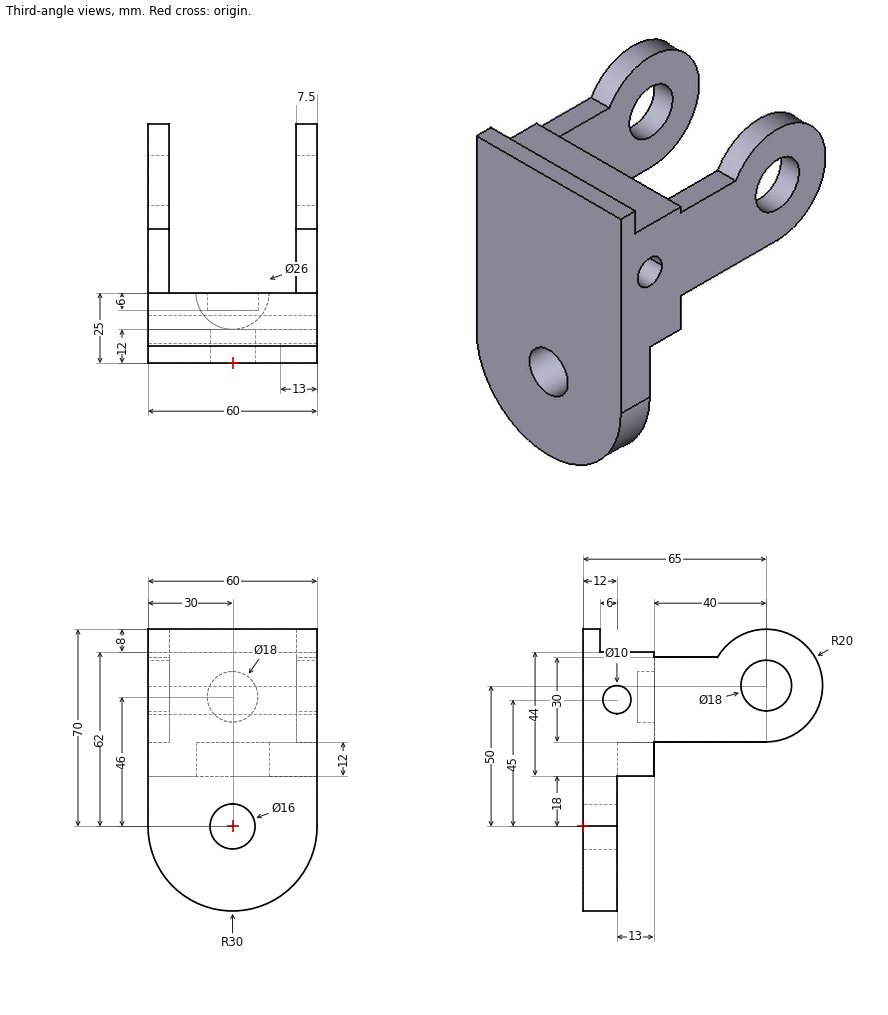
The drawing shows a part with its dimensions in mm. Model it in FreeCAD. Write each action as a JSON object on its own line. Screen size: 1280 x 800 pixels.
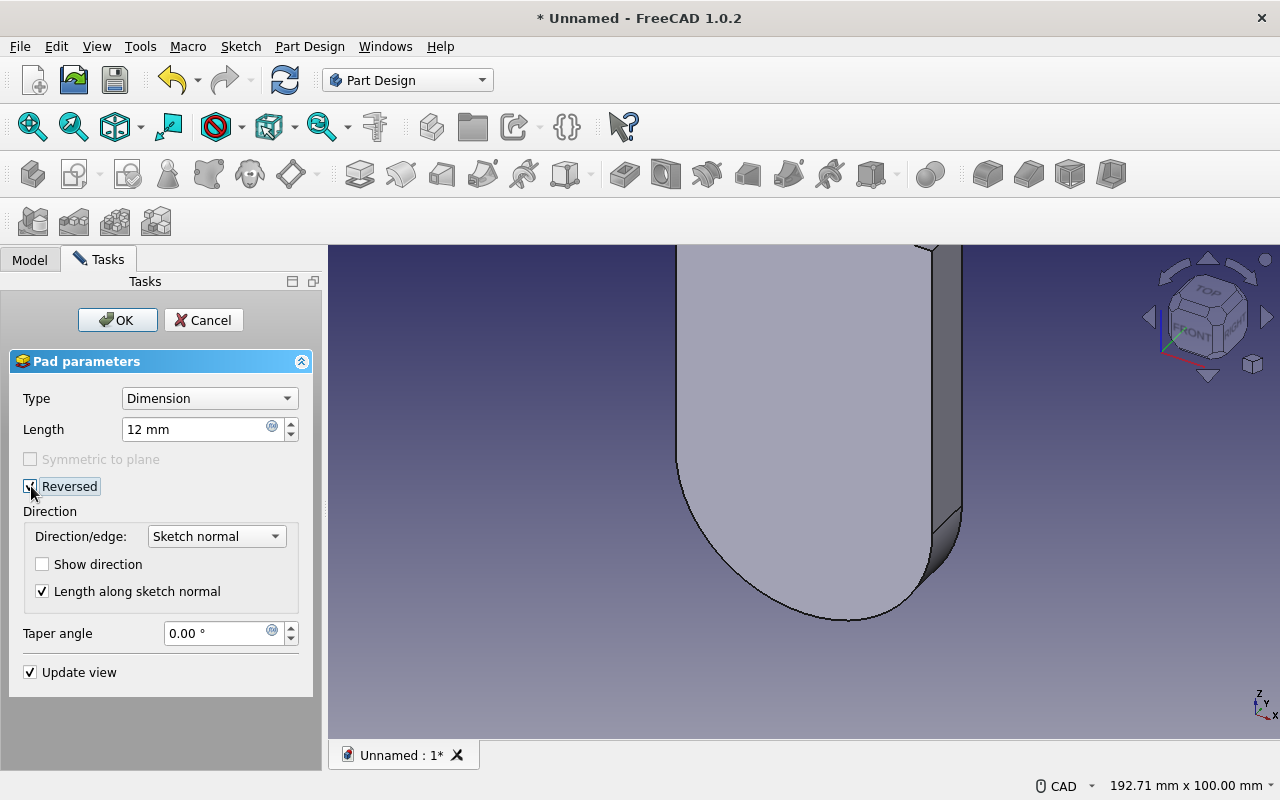
{"action": "left_click", "coordinate": [118, 320]}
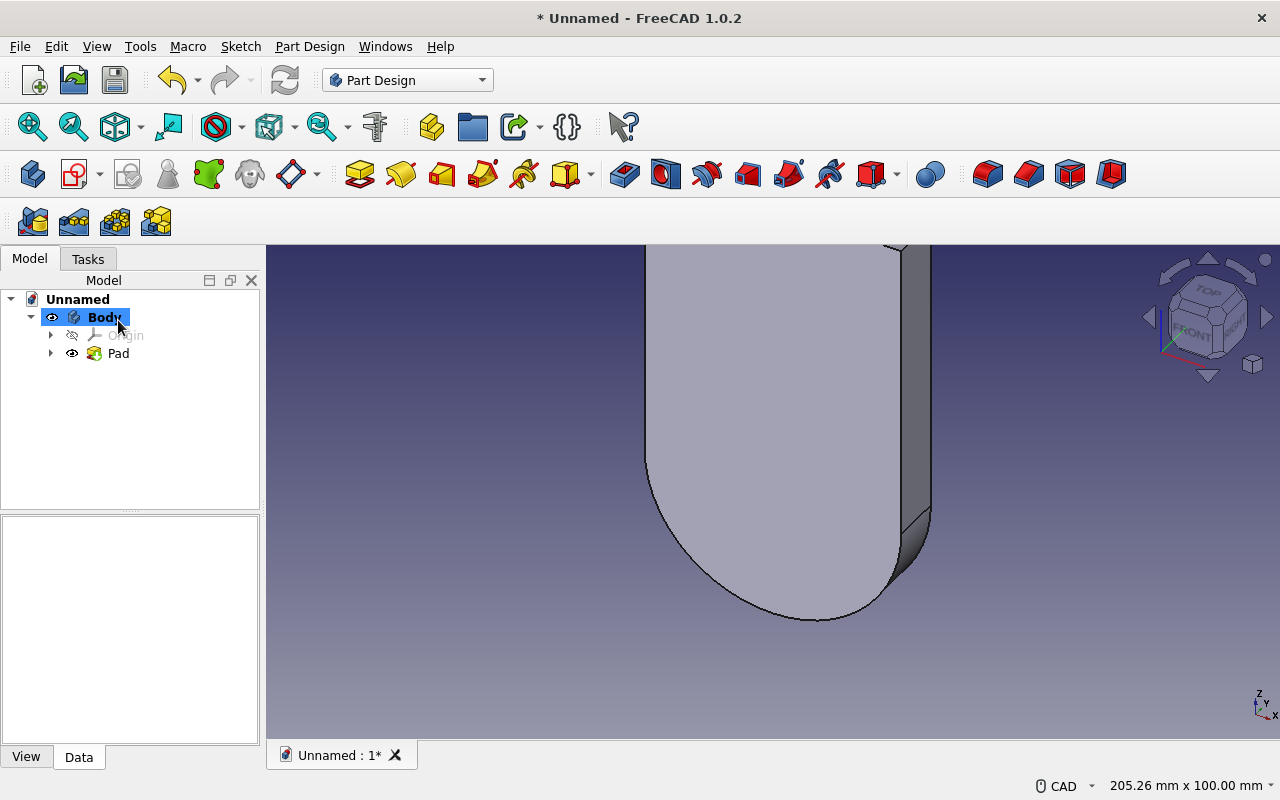
{"action": "key", "text": "v f"}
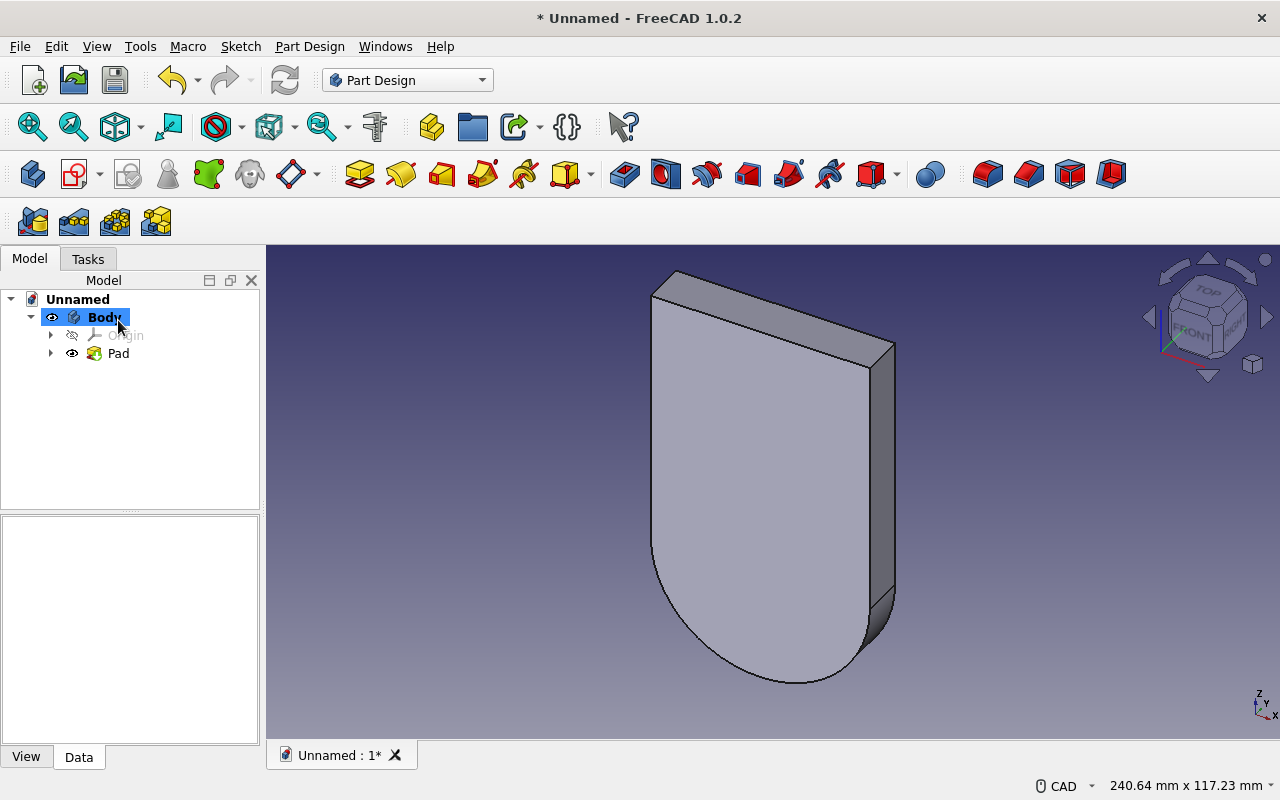
{"action": "key", "text": "4"}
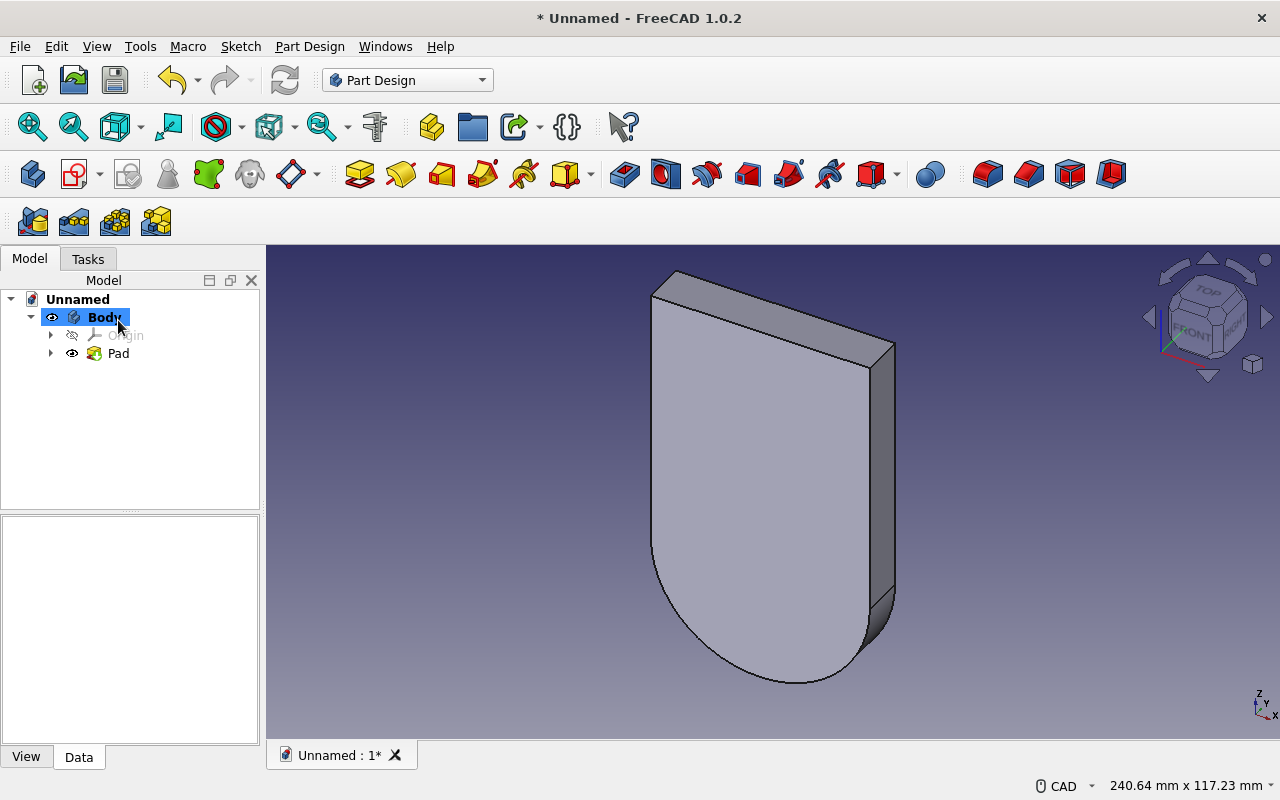
{"action": "left_click", "coordinate": [773, 431]}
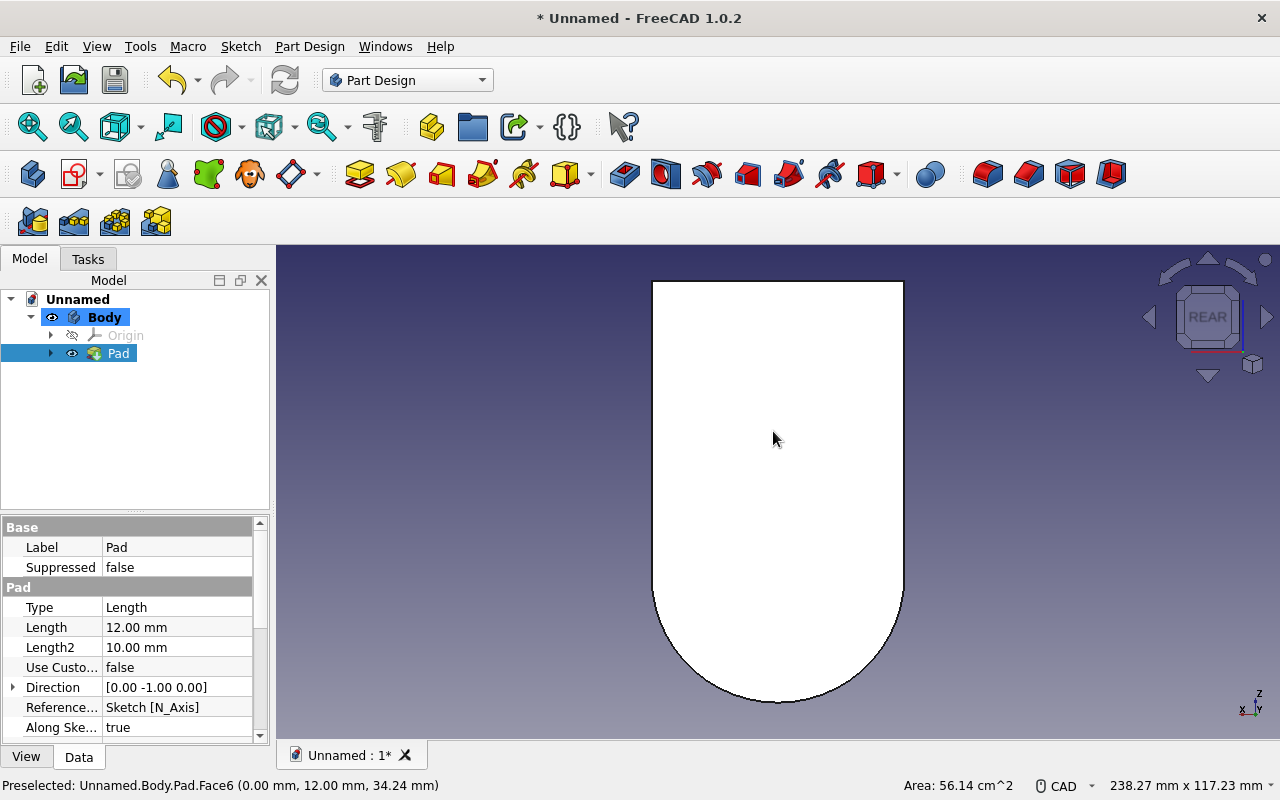
{"action": "left_click", "coordinate": [74, 174]}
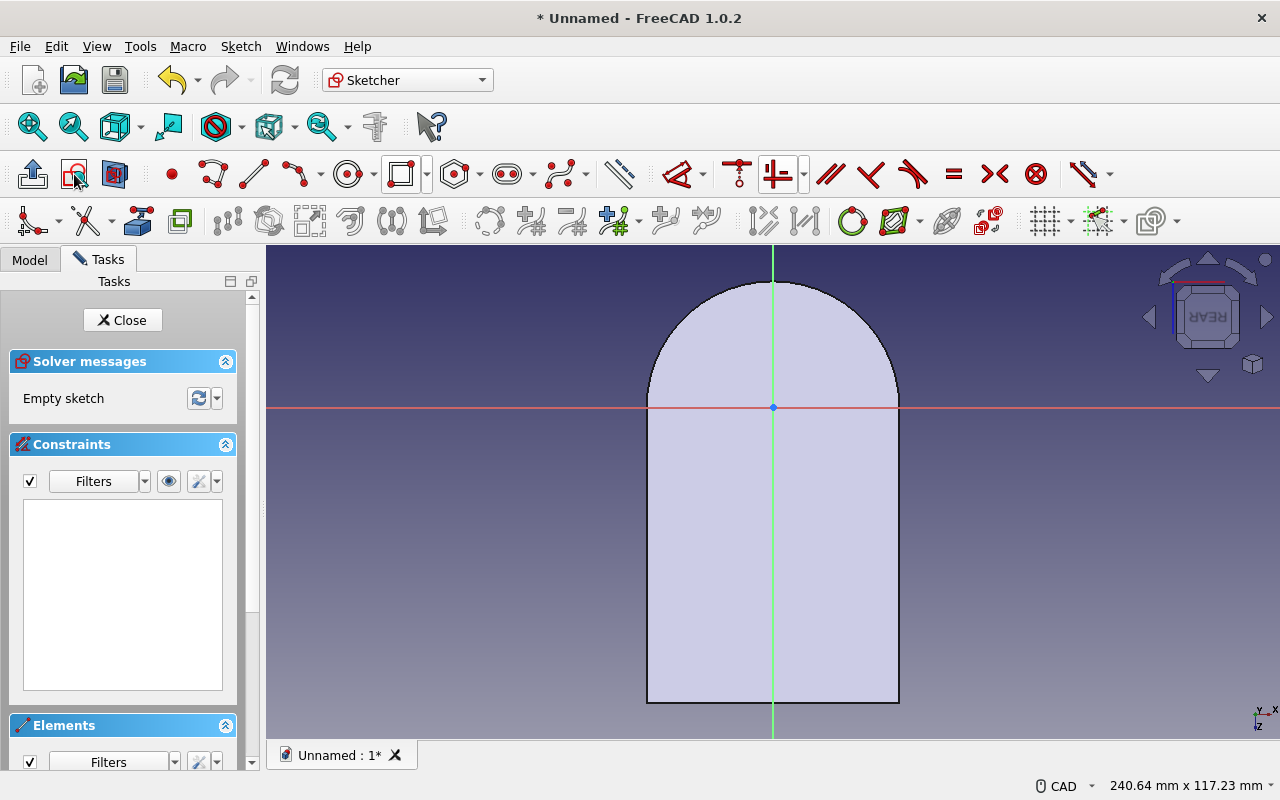
{"action": "scroll", "coordinate": [790, 386], "scroll_direction": "up", "scroll_amount": 8}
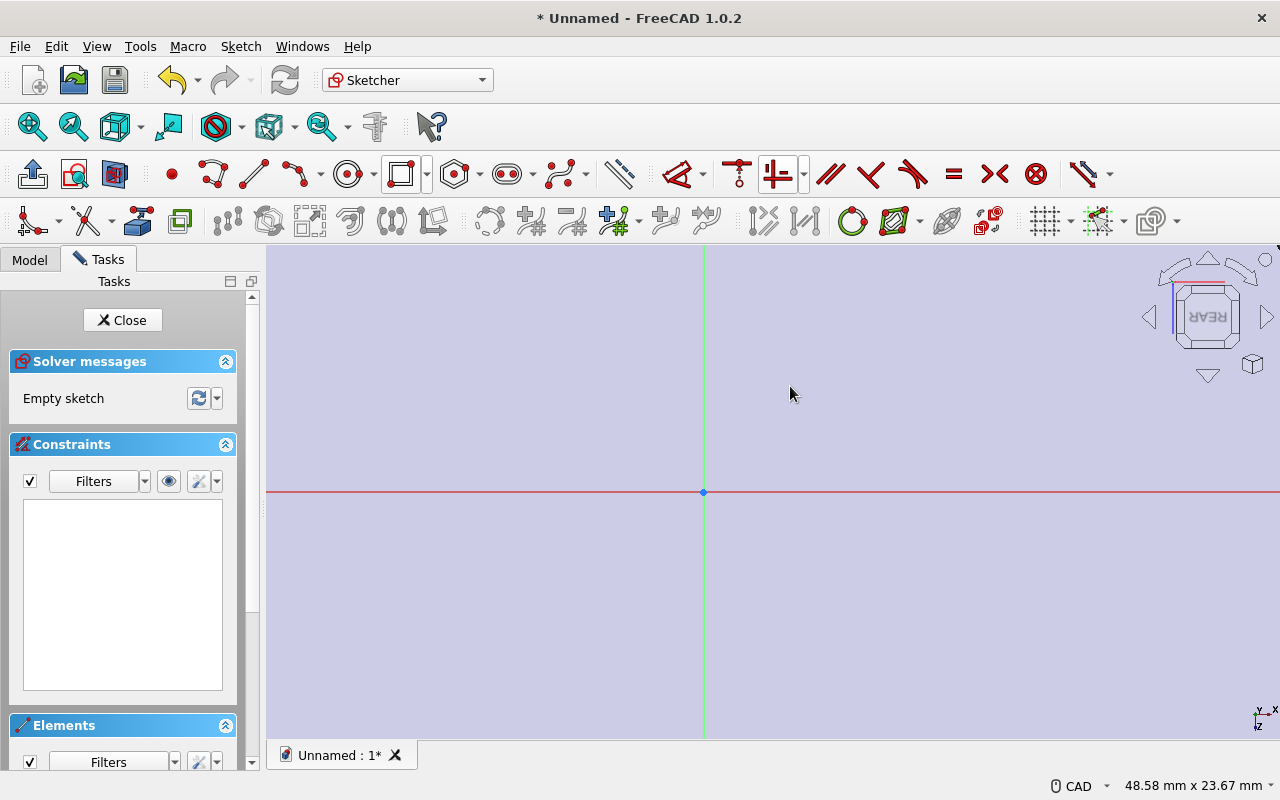
{"action": "key", "text": "g c"}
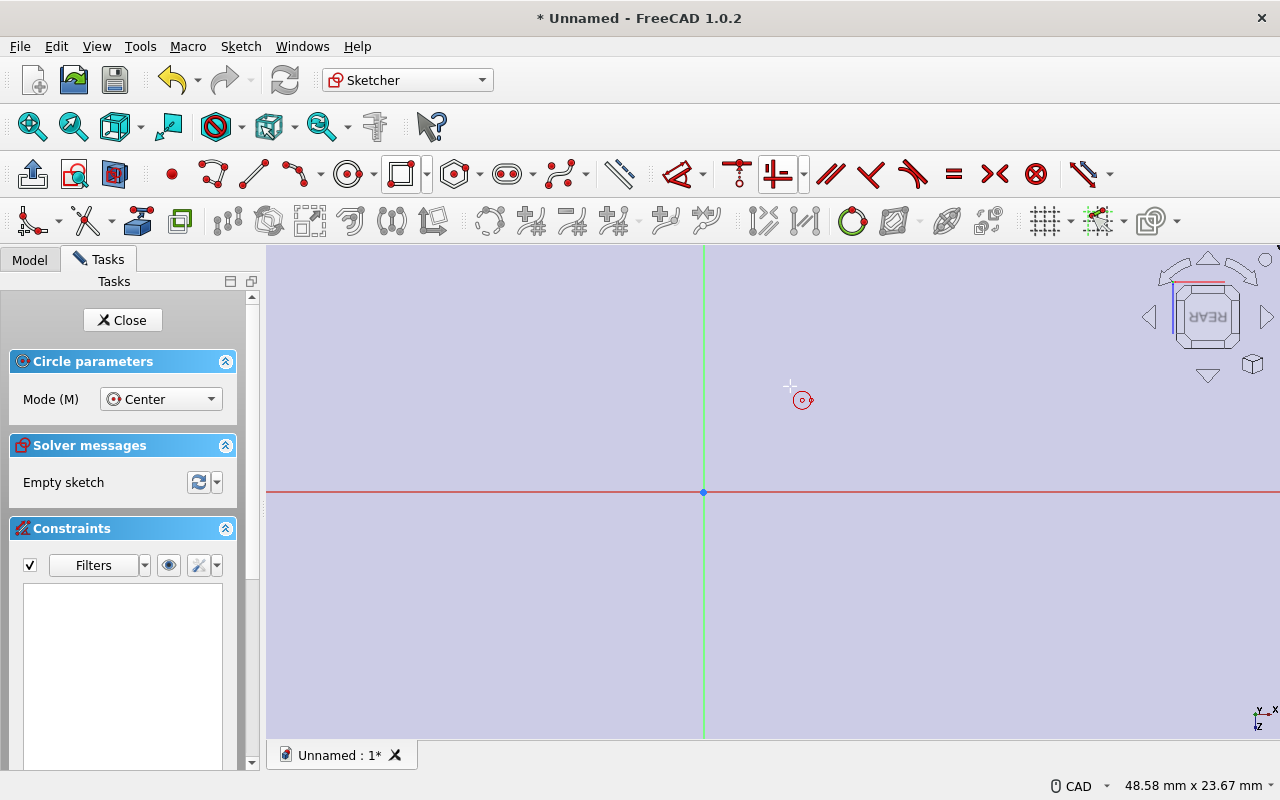
{"action": "left_click", "coordinate": [704, 492]}
{"action": "left_click", "coordinate": [822, 374]}
{"action": "key", "text": "Escape"}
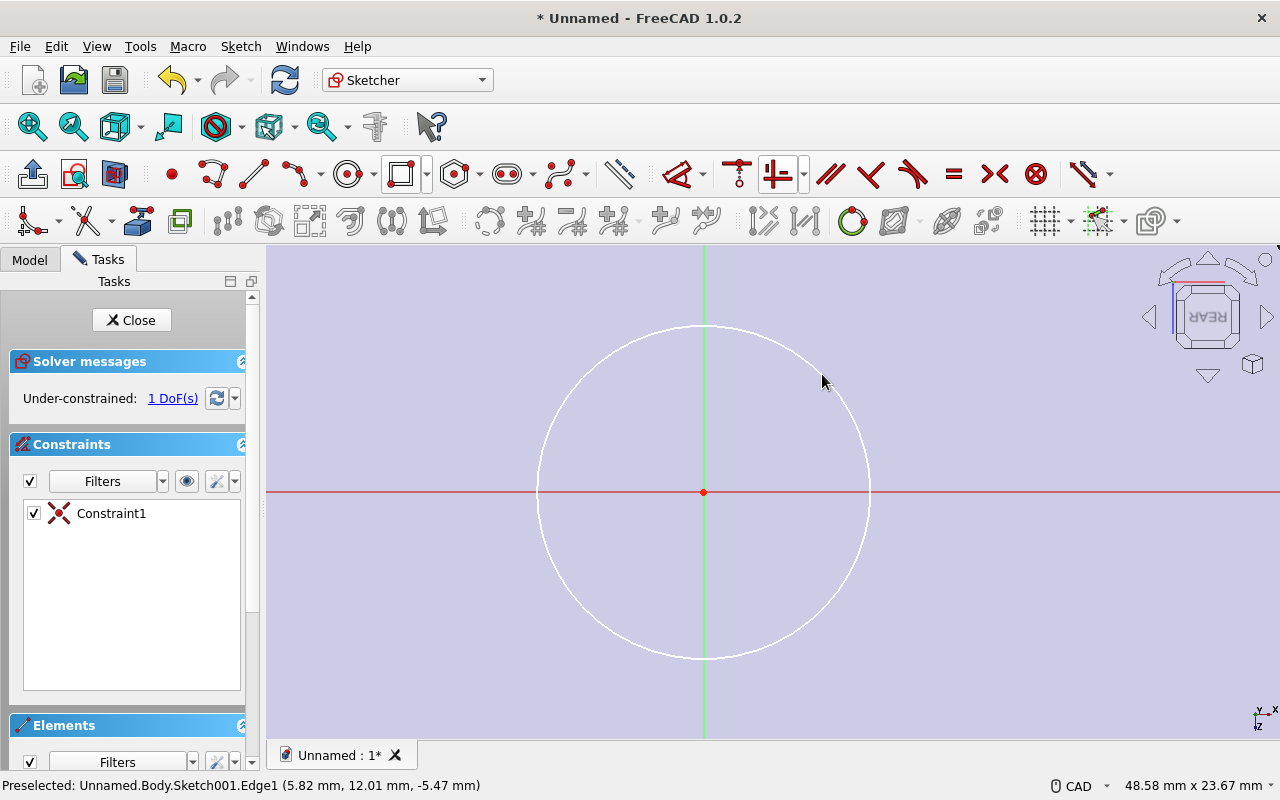
{"action": "left_click", "coordinate": [676, 174]}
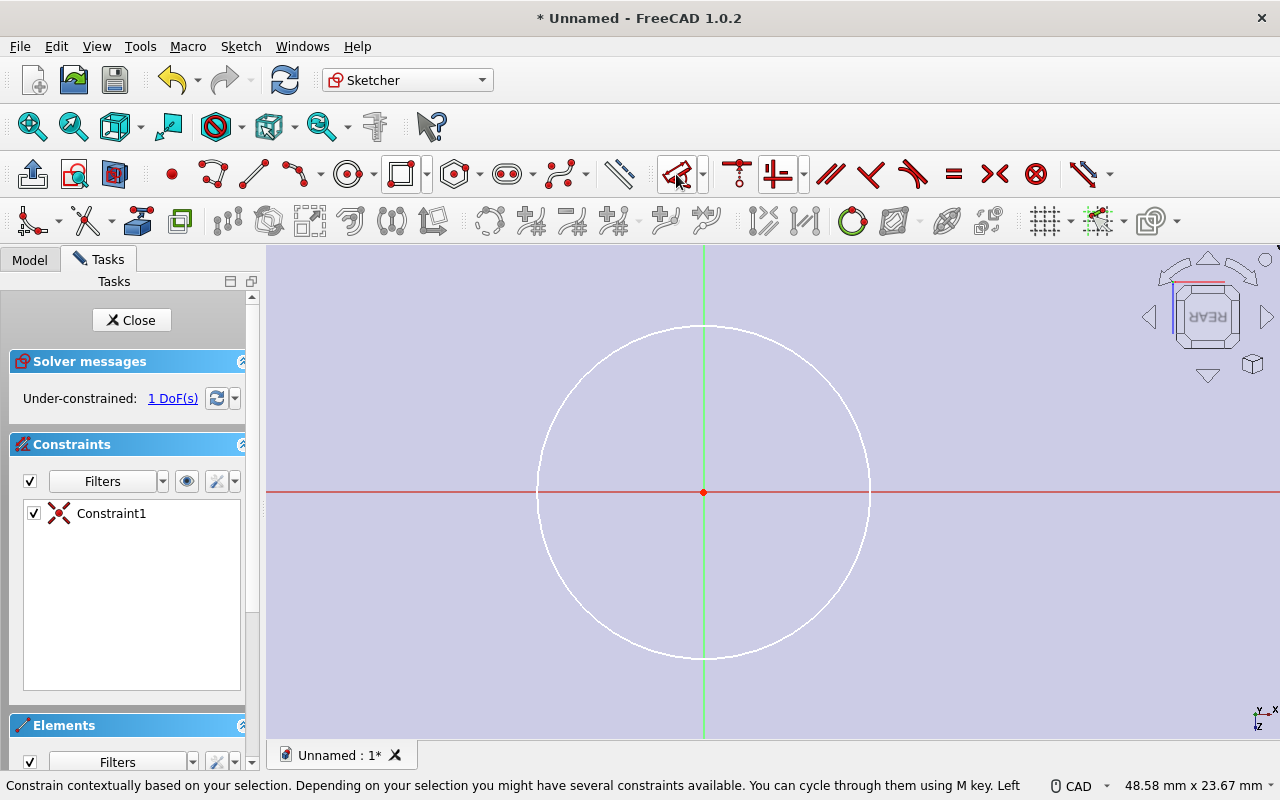
{"action": "left_click", "coordinate": [821, 374]}
{"action": "left_click", "coordinate": [844, 351]}